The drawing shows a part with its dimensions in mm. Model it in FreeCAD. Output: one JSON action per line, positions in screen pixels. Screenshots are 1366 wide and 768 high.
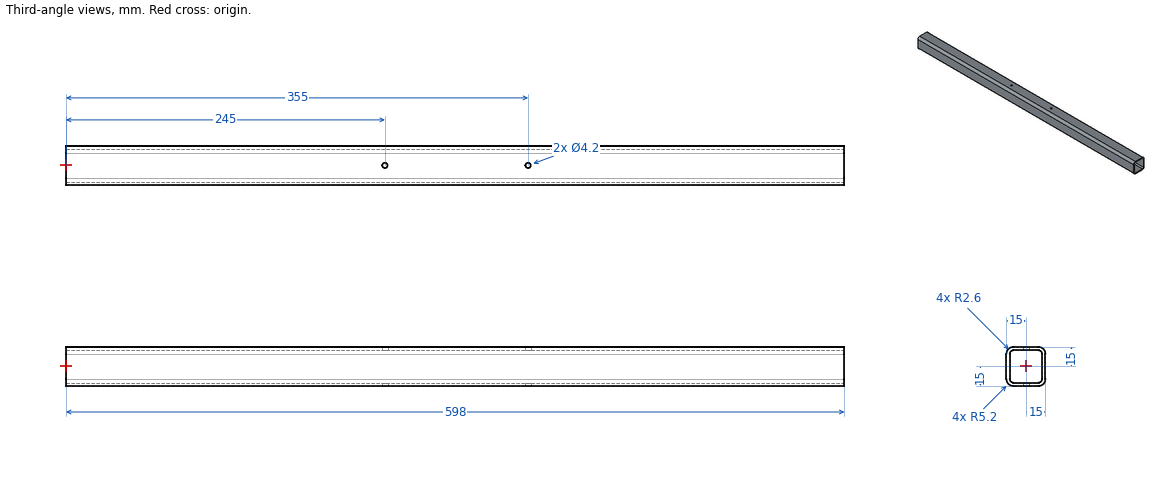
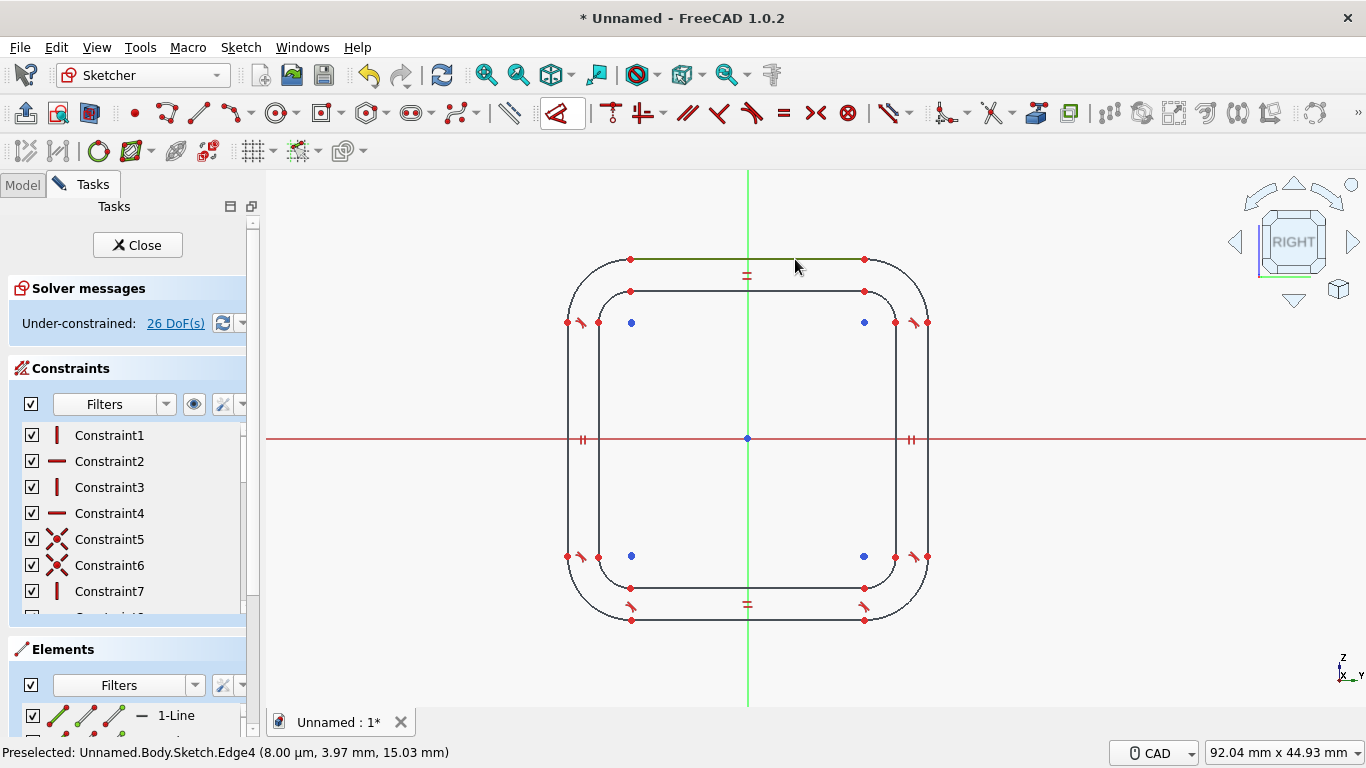
{"action": "left_click", "coordinate": [921, 294]}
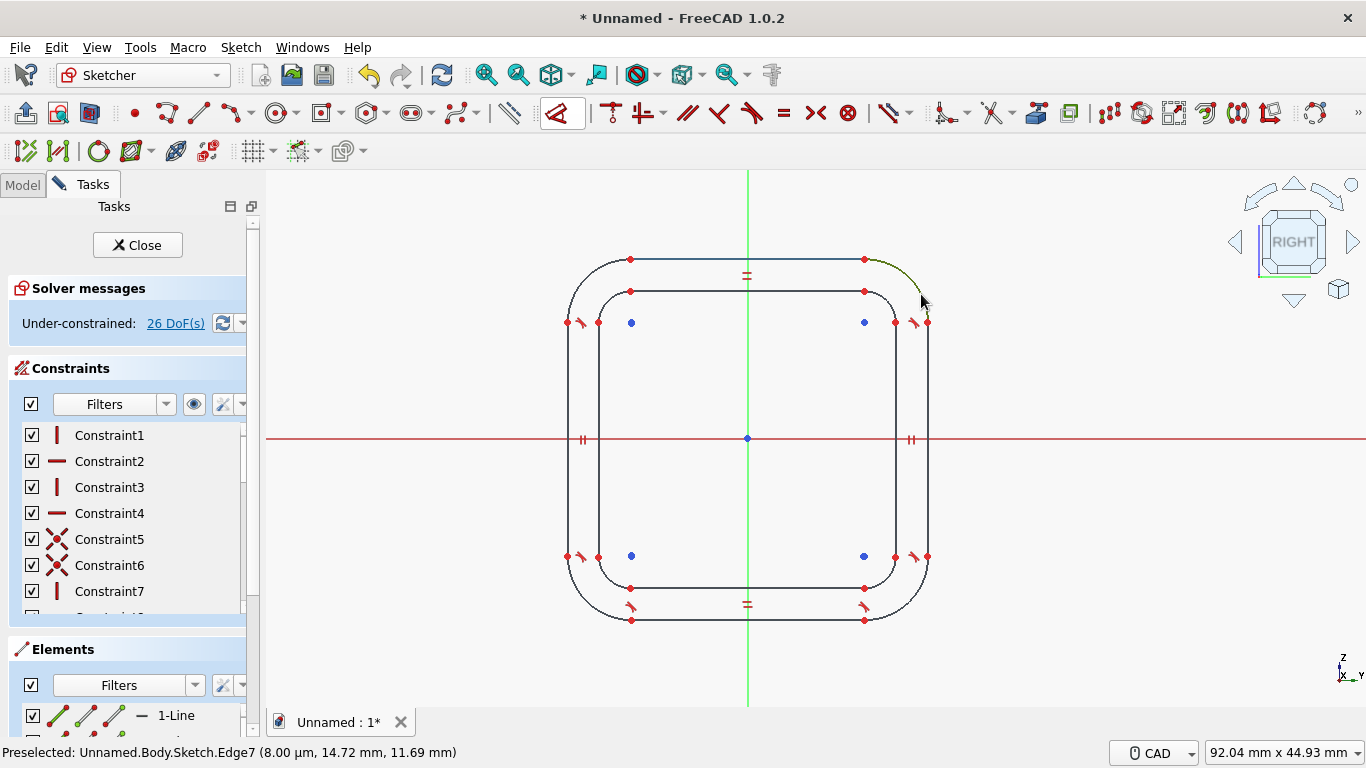
{"action": "key", "text": "t"}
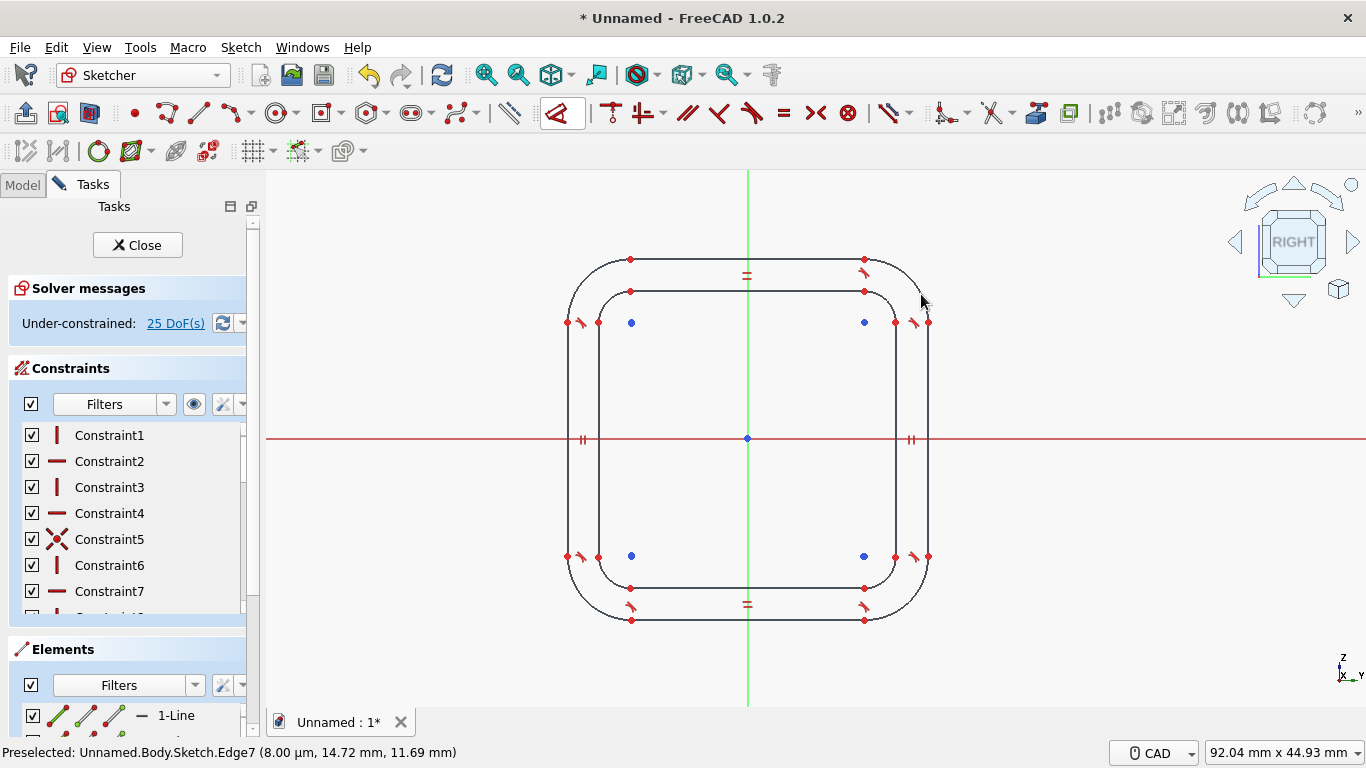
{"action": "left_click", "coordinate": [795, 259]}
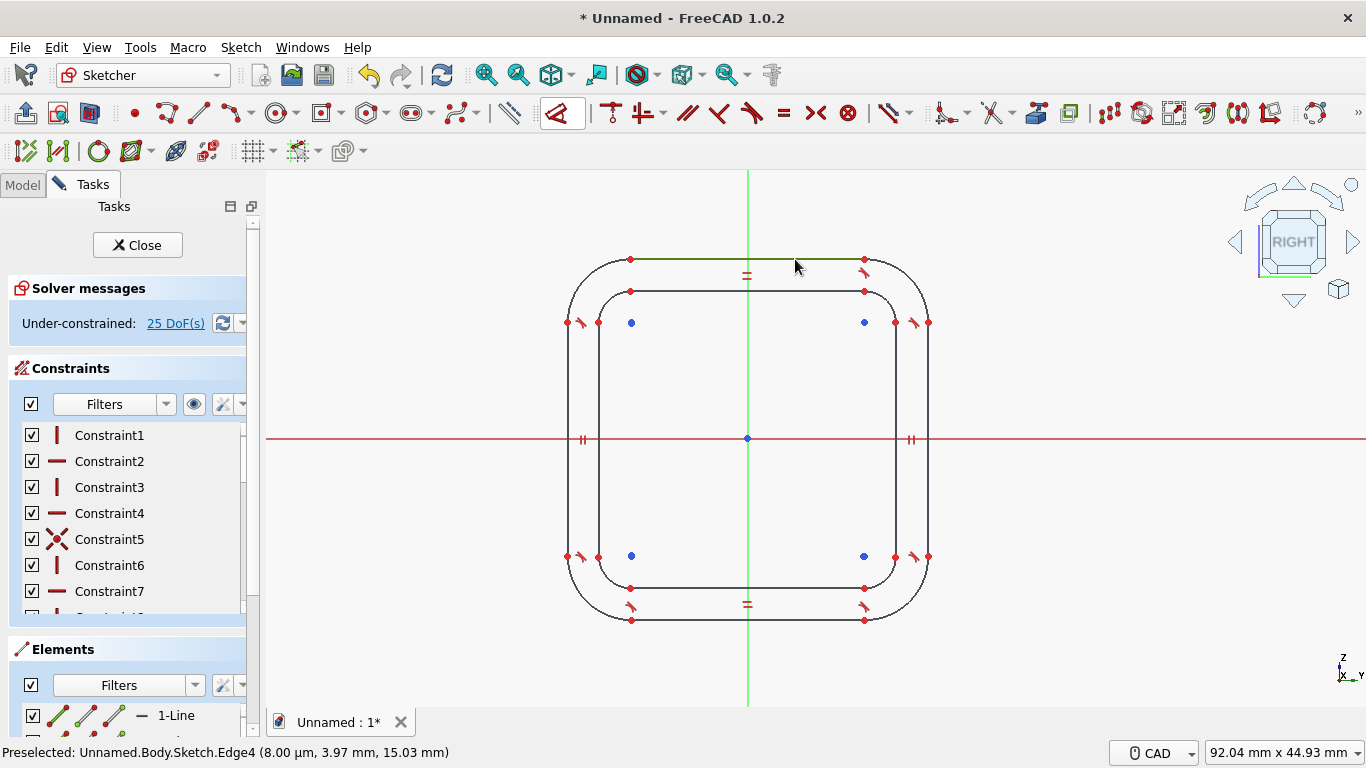
{"action": "left_click", "coordinate": [602, 266]}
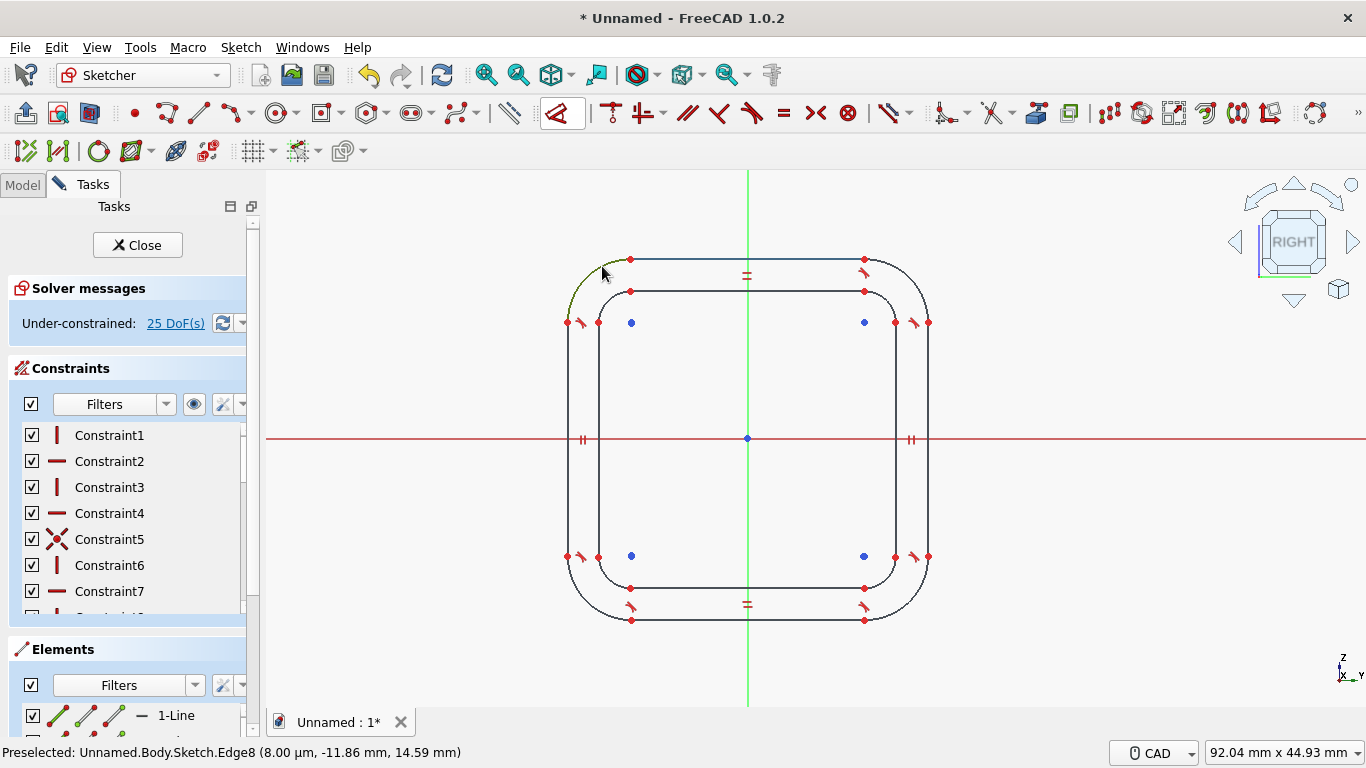
{"action": "left_click", "coordinate": [752, 114]}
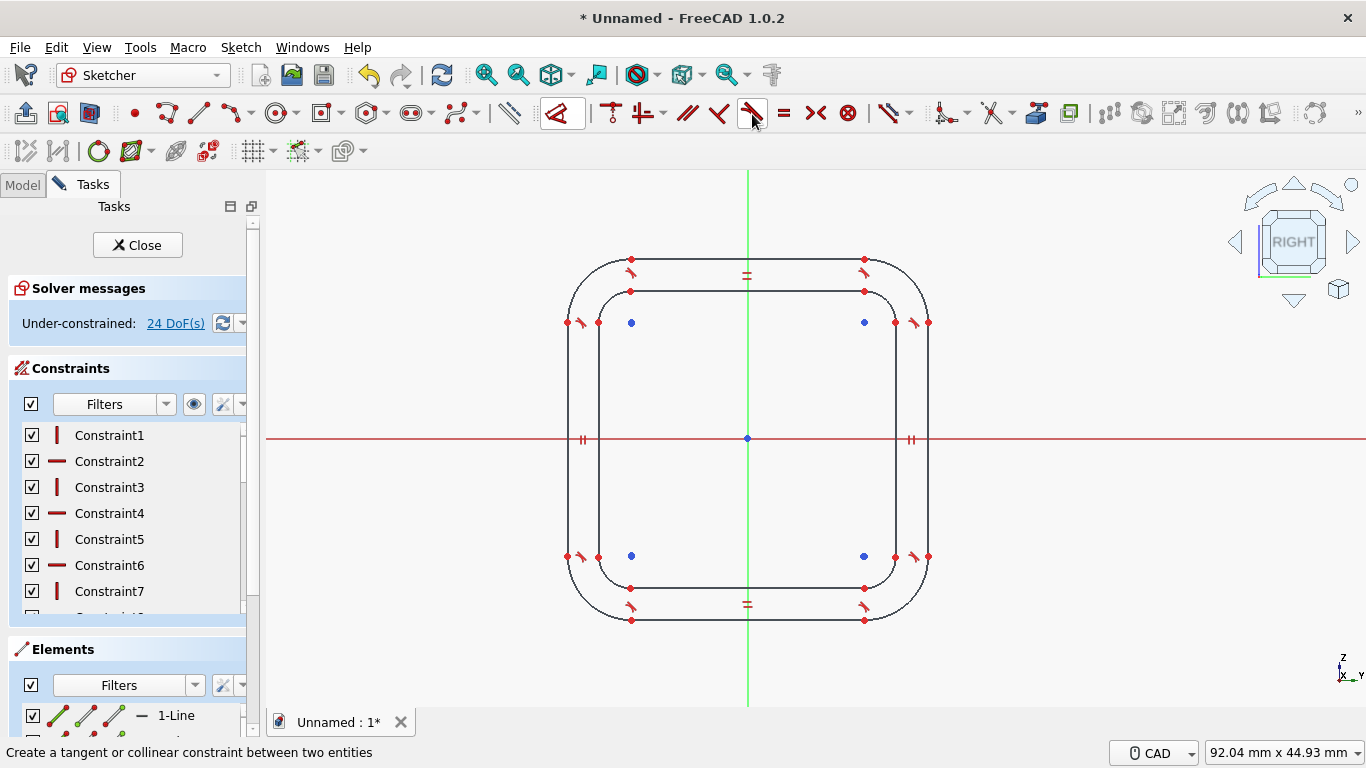
{"action": "left_click", "coordinate": [599, 487]}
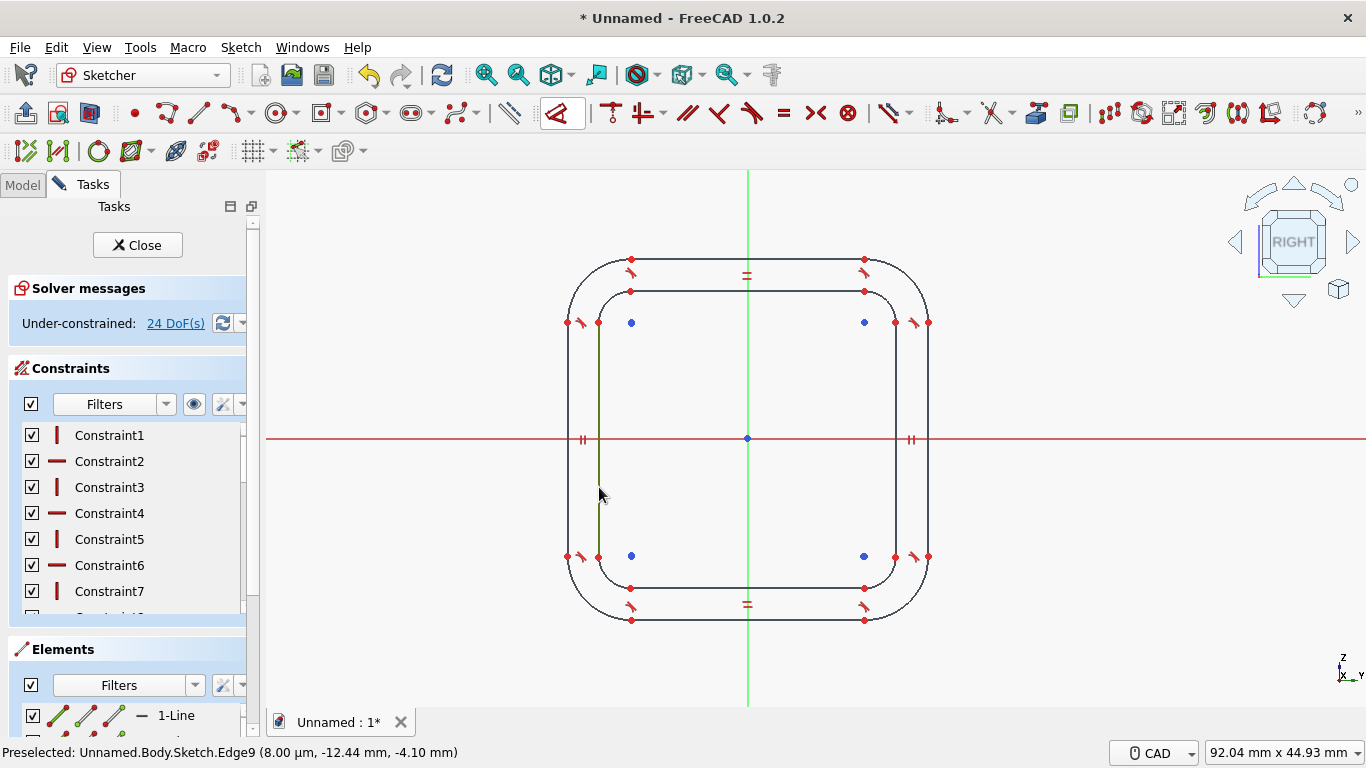
{"action": "left_click", "coordinate": [617, 295]}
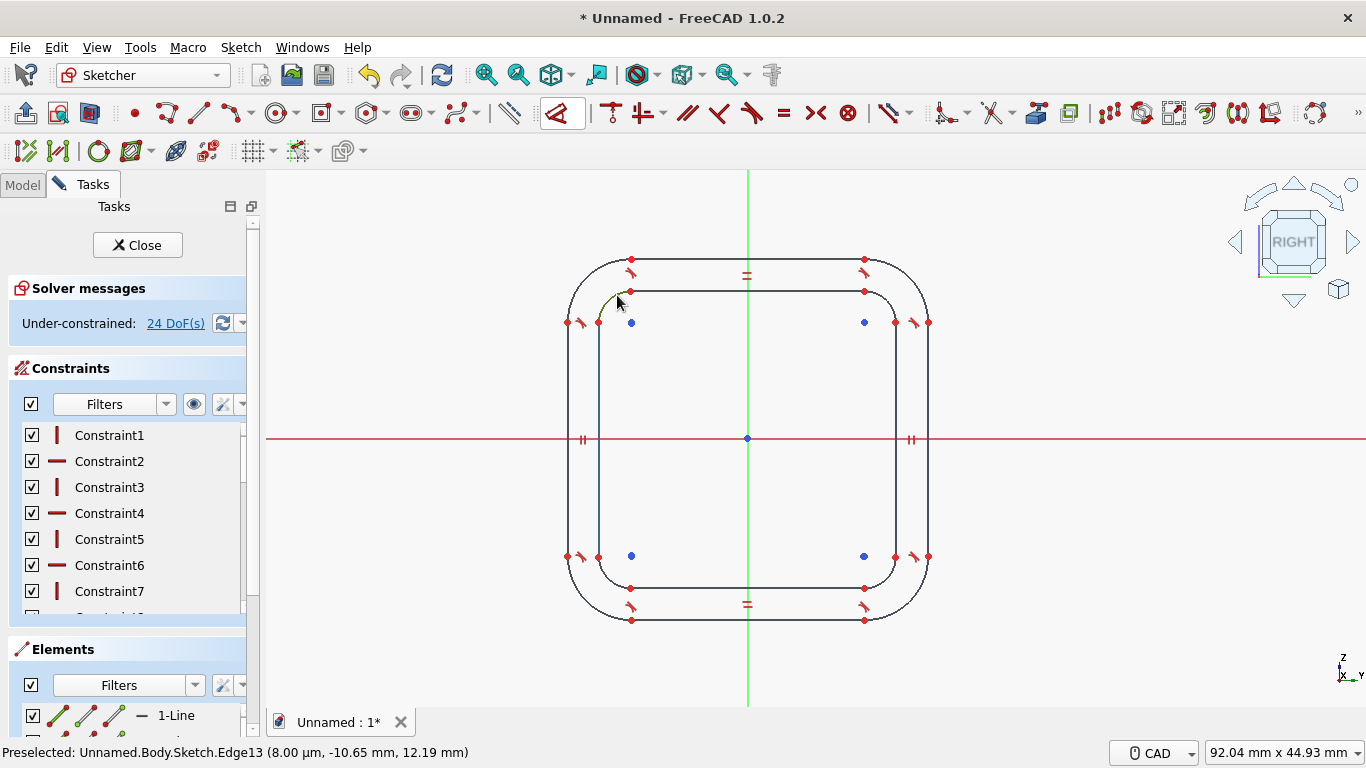
{"action": "key", "text": "t"}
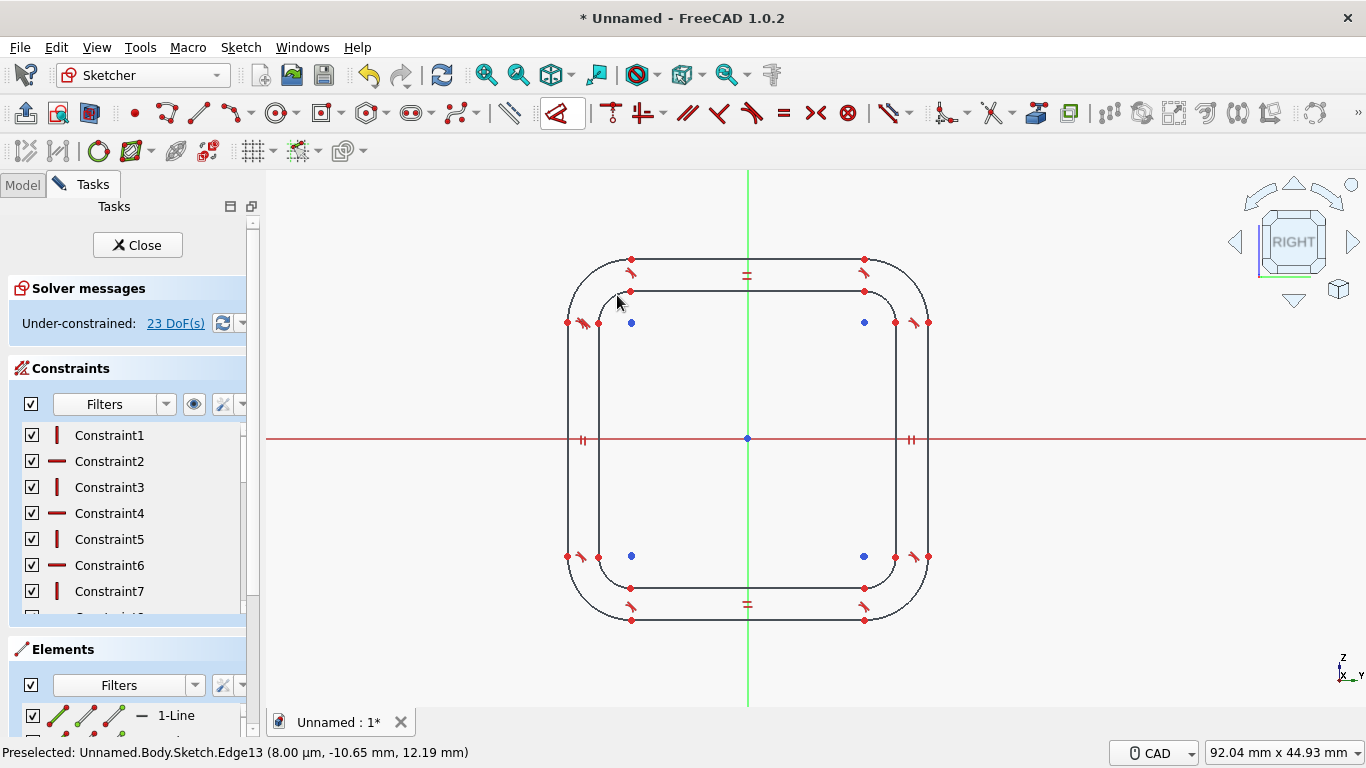
{"action": "left_click", "coordinate": [599, 487]}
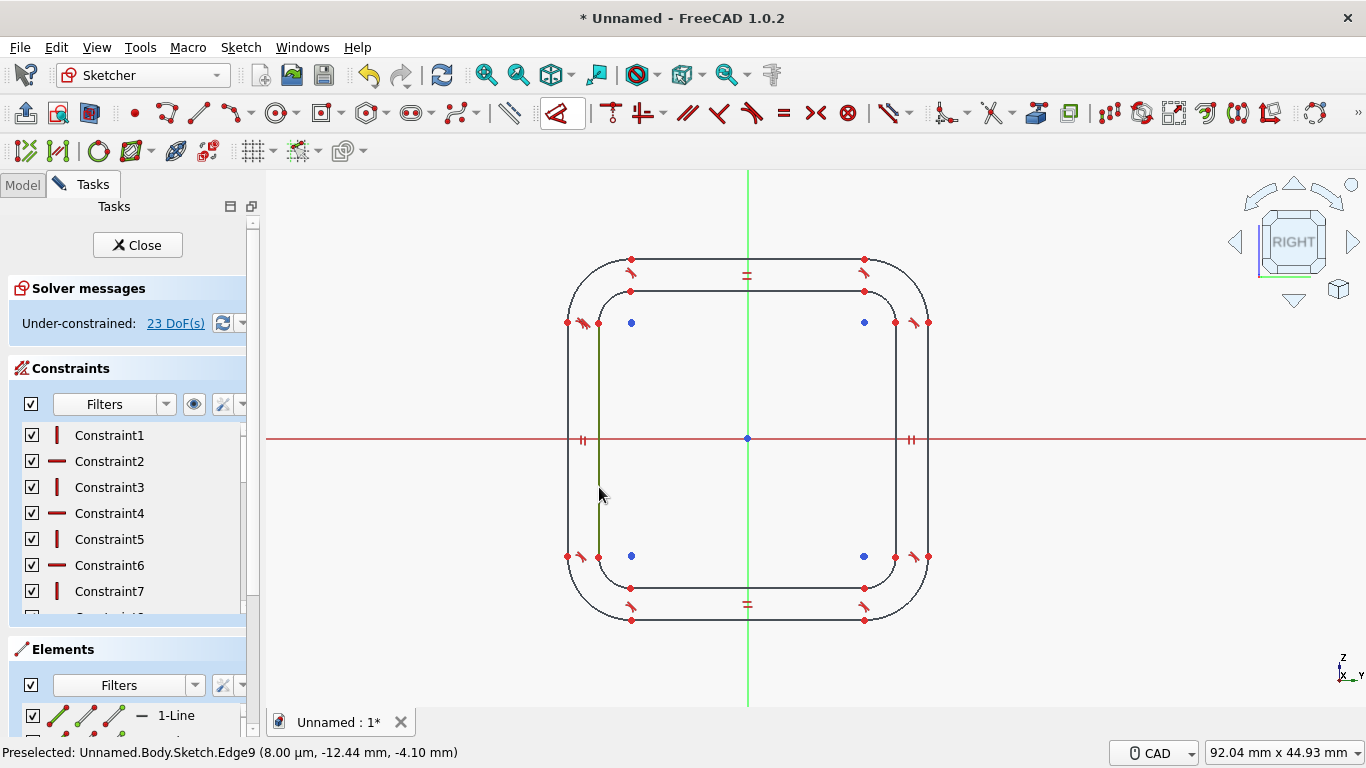
{"action": "left_click", "coordinate": [603, 571]}